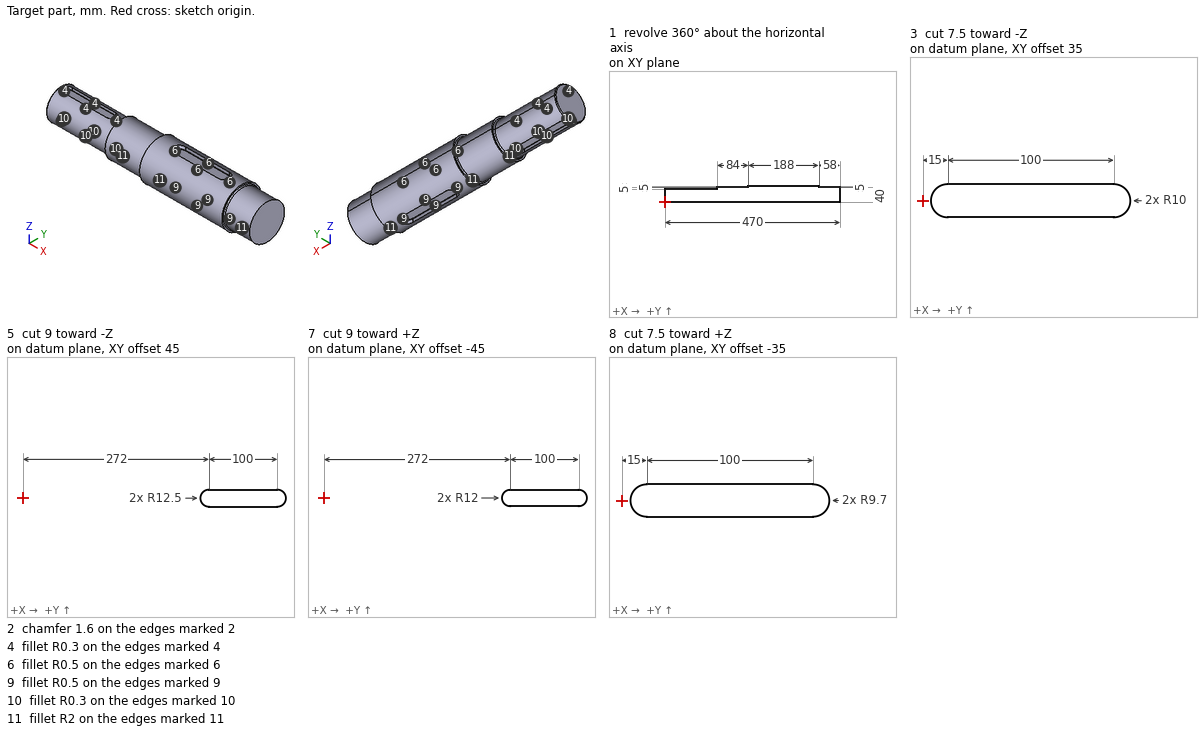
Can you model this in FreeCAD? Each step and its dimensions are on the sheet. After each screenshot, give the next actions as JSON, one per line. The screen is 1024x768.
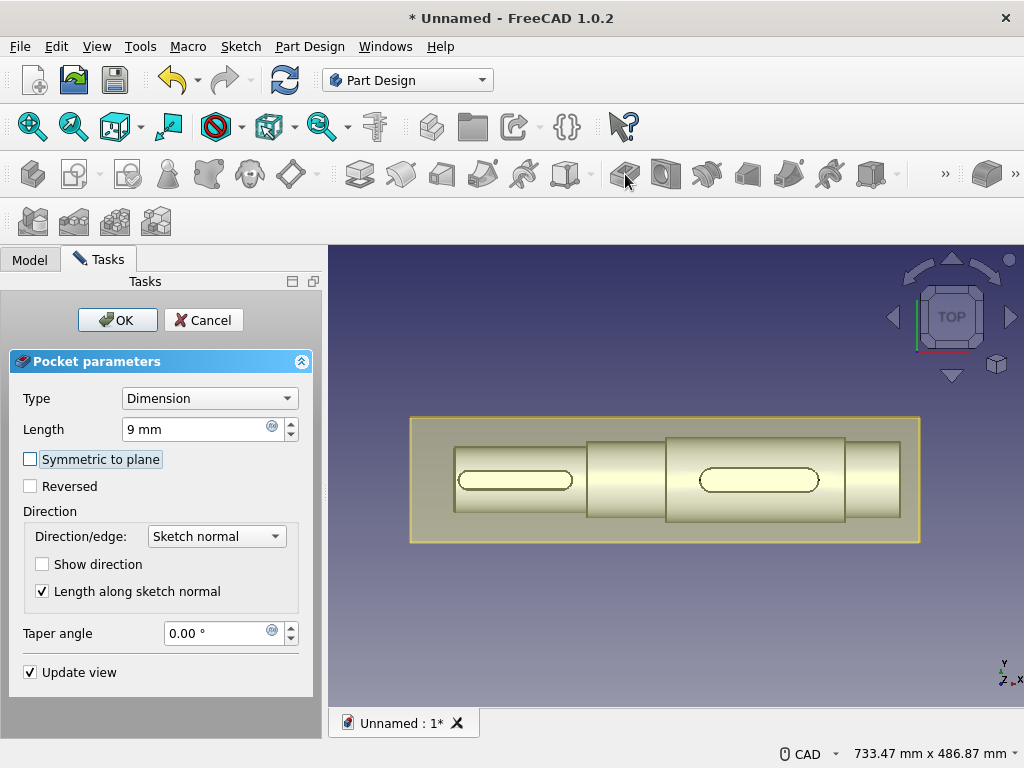
{"action": "left_click", "coordinate": [118, 320]}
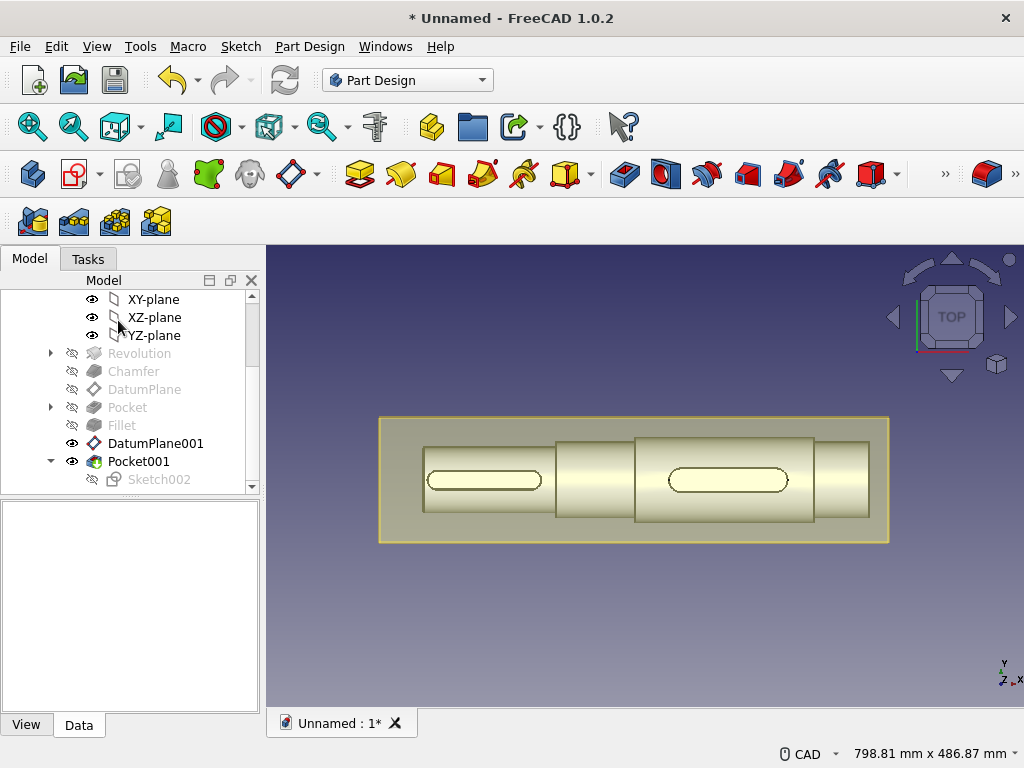
{"action": "left_click", "coordinate": [117, 443]}
{"action": "key", "text": "space"}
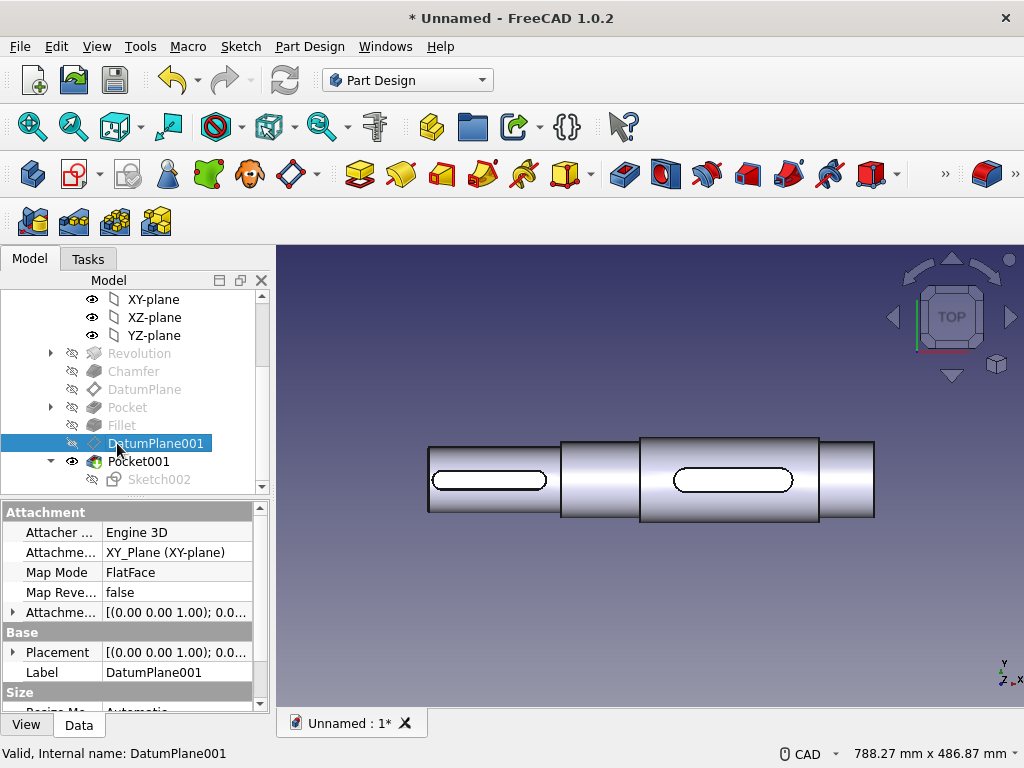
{"action": "left_click", "coordinate": [767, 479]}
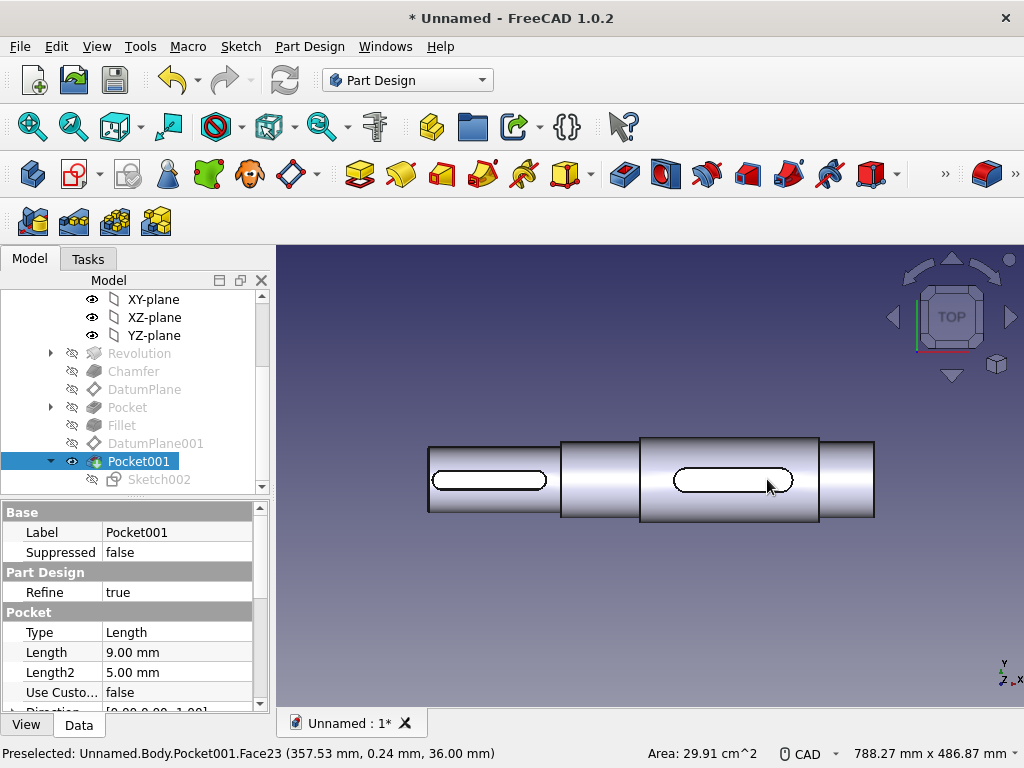
{"action": "left_click", "coordinate": [987, 174]}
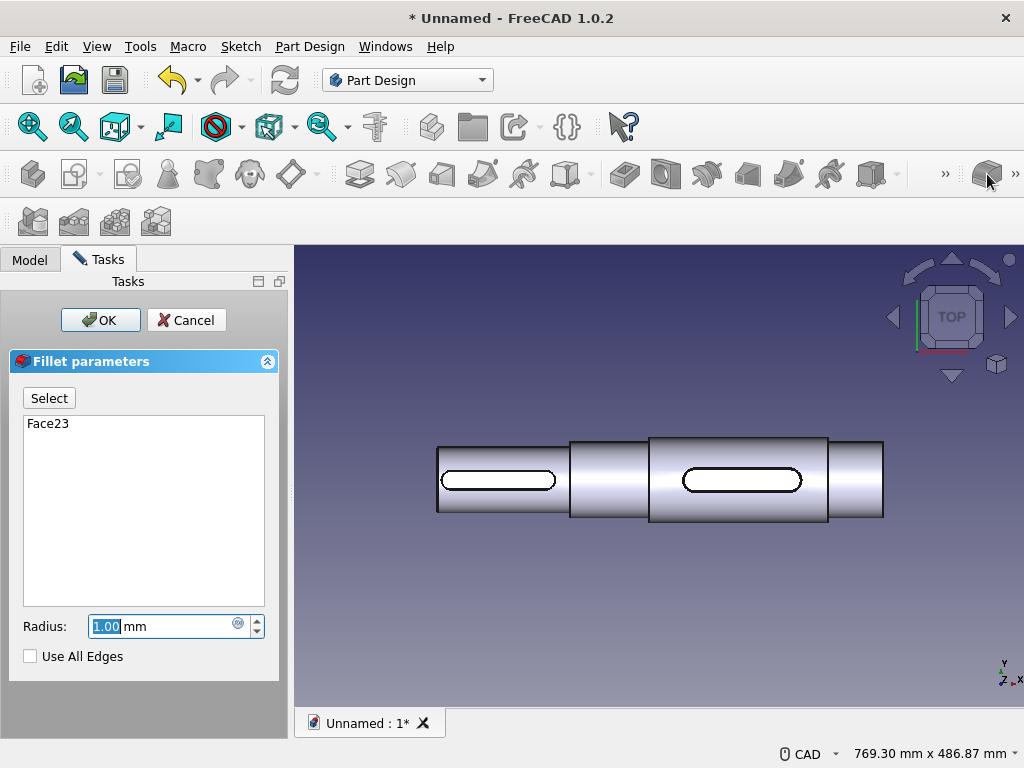
{"action": "type", "text": "0.5"}
{"action": "key", "text": "Tab"}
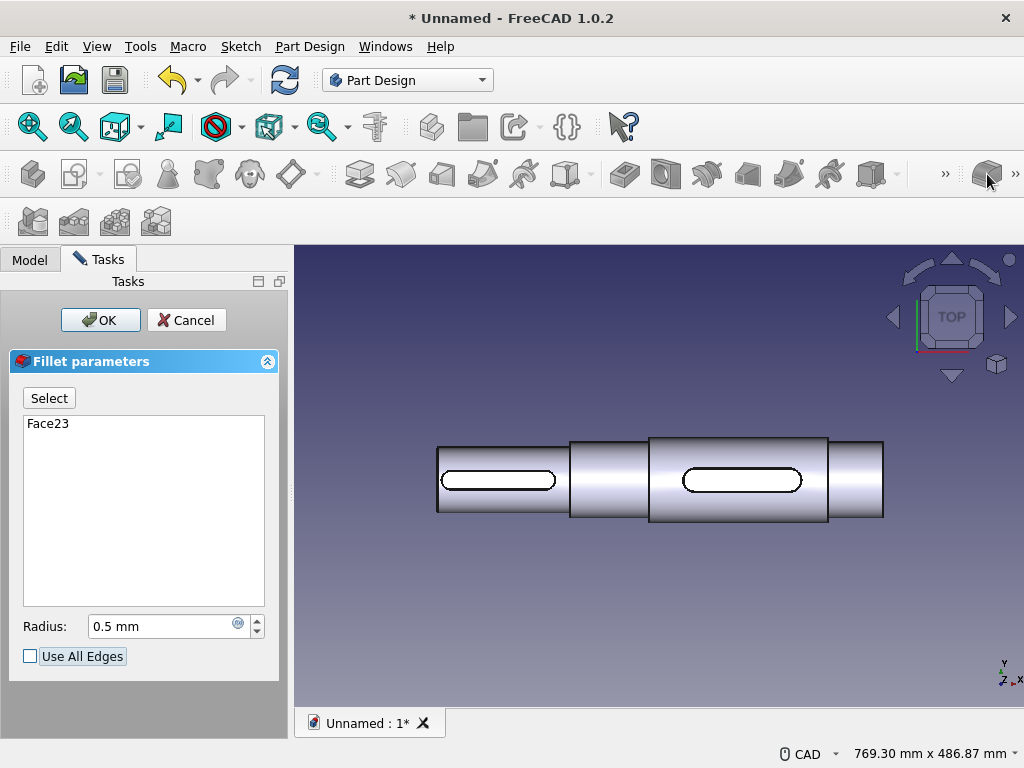
{"action": "left_click", "coordinate": [101, 320]}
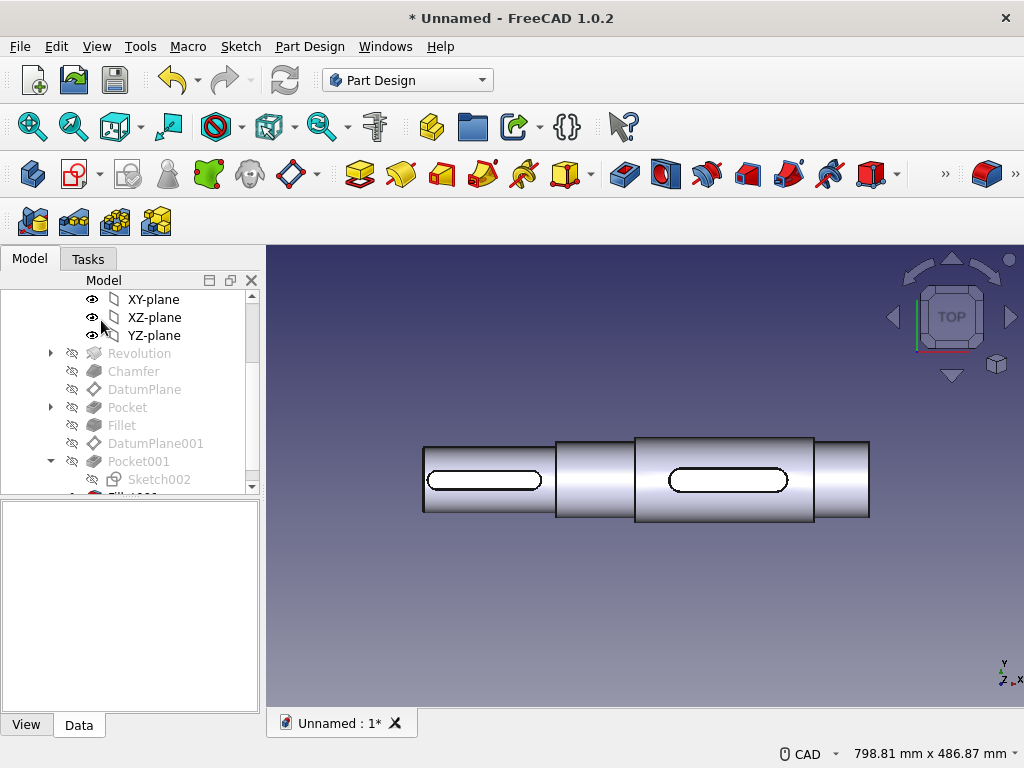
{"action": "scroll", "coordinate": [161, 385], "scroll_direction": "down", "scroll_amount": 3}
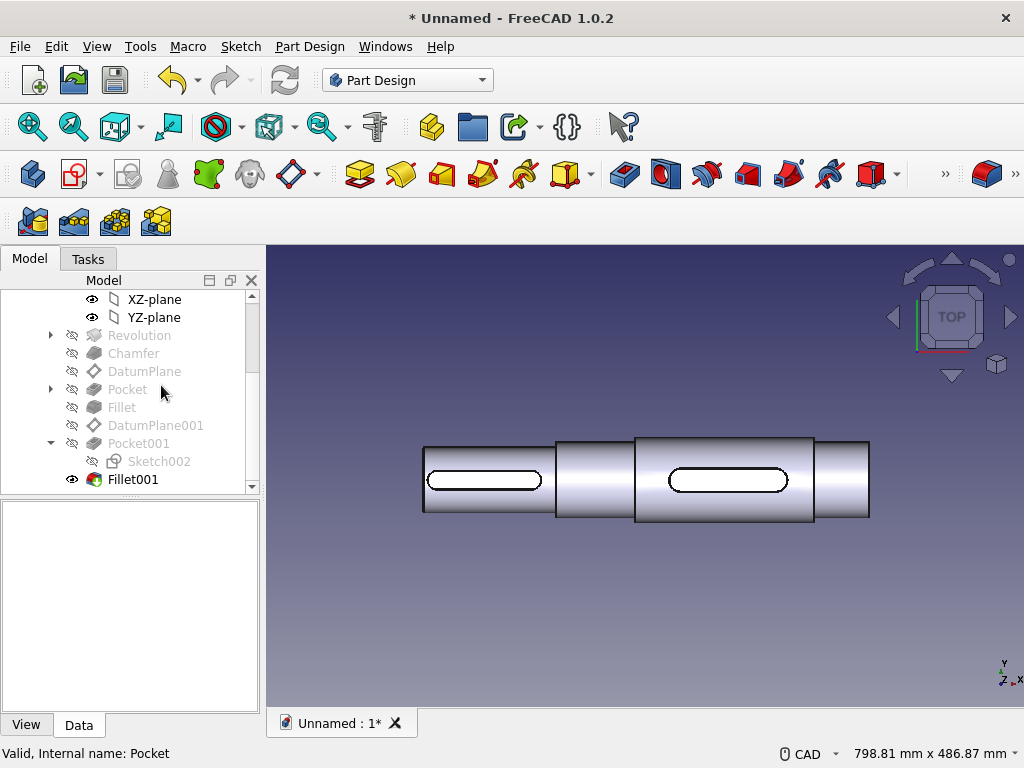
{"action": "scroll", "coordinate": [161, 385], "scroll_direction": "up", "scroll_amount": 15}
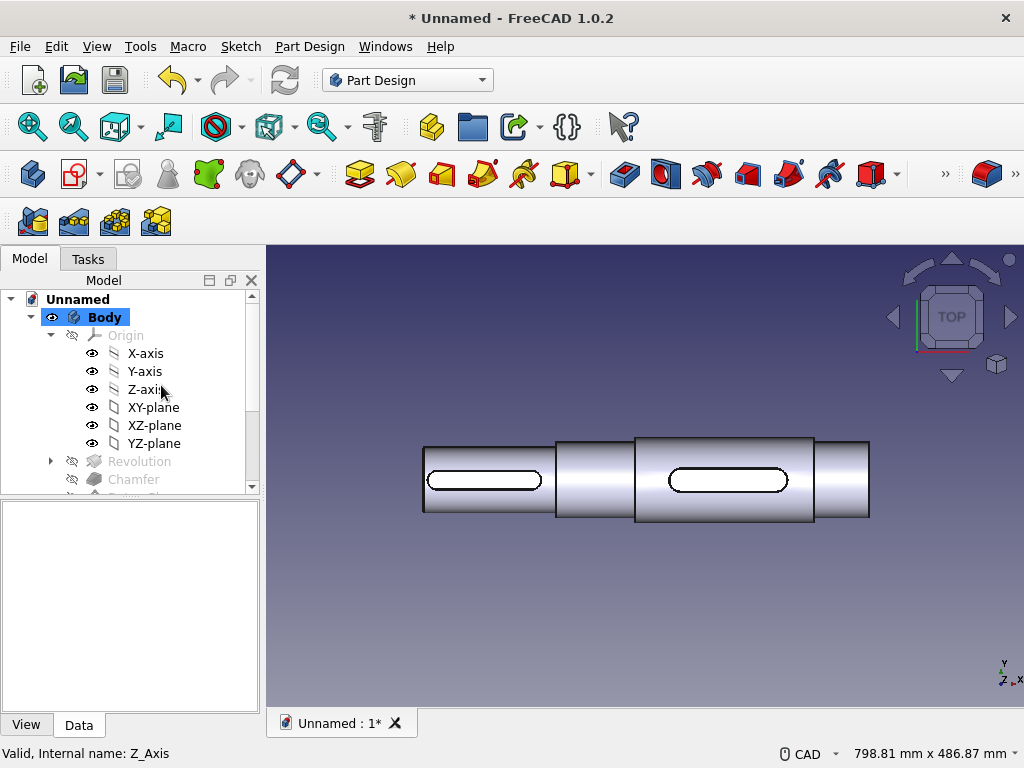
{"action": "left_click", "coordinate": [137, 407]}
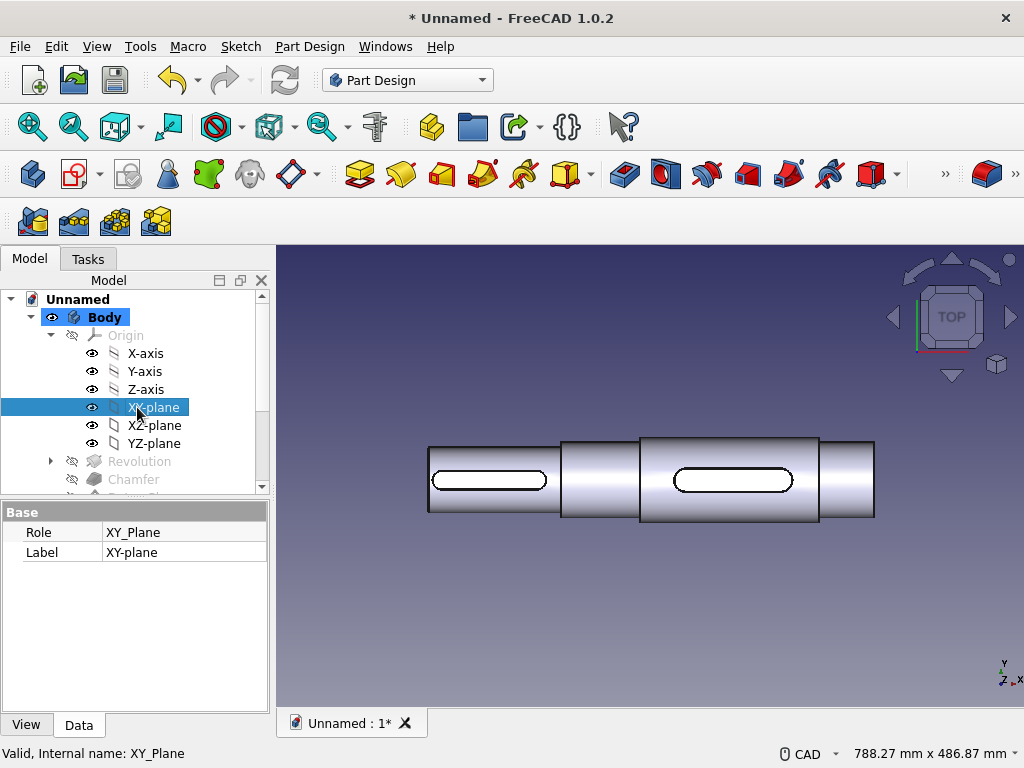
{"action": "left_click", "coordinate": [290, 174]}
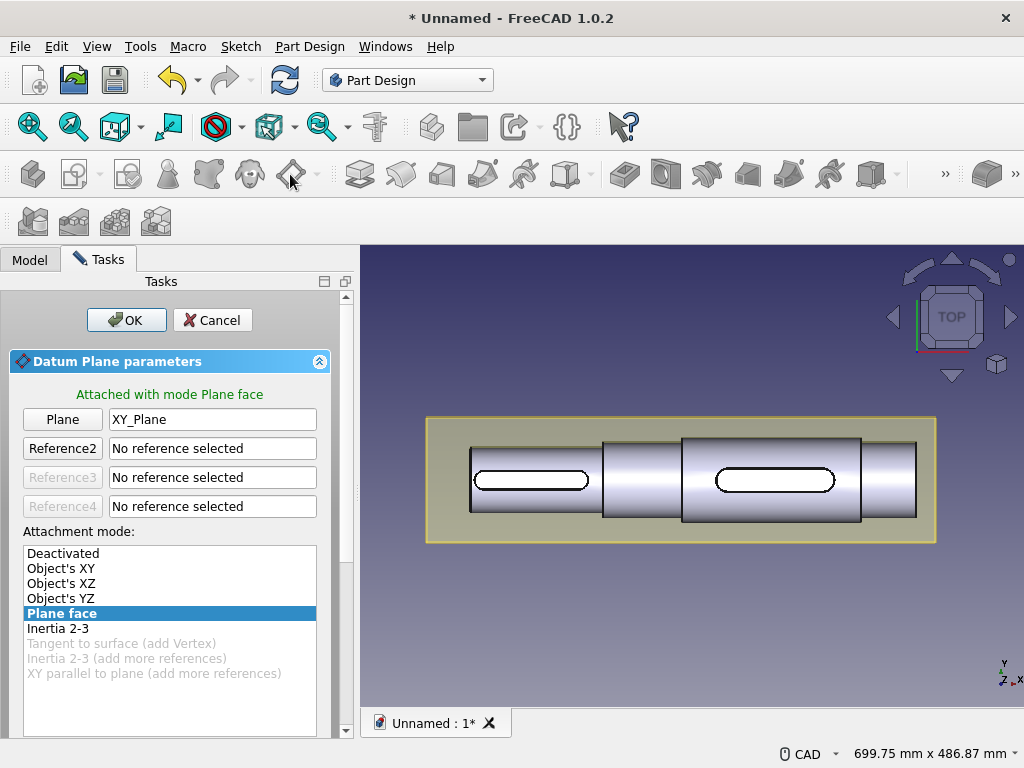
{"action": "scroll", "coordinate": [346, 514], "scroll_direction": "down", "scroll_amount": 4}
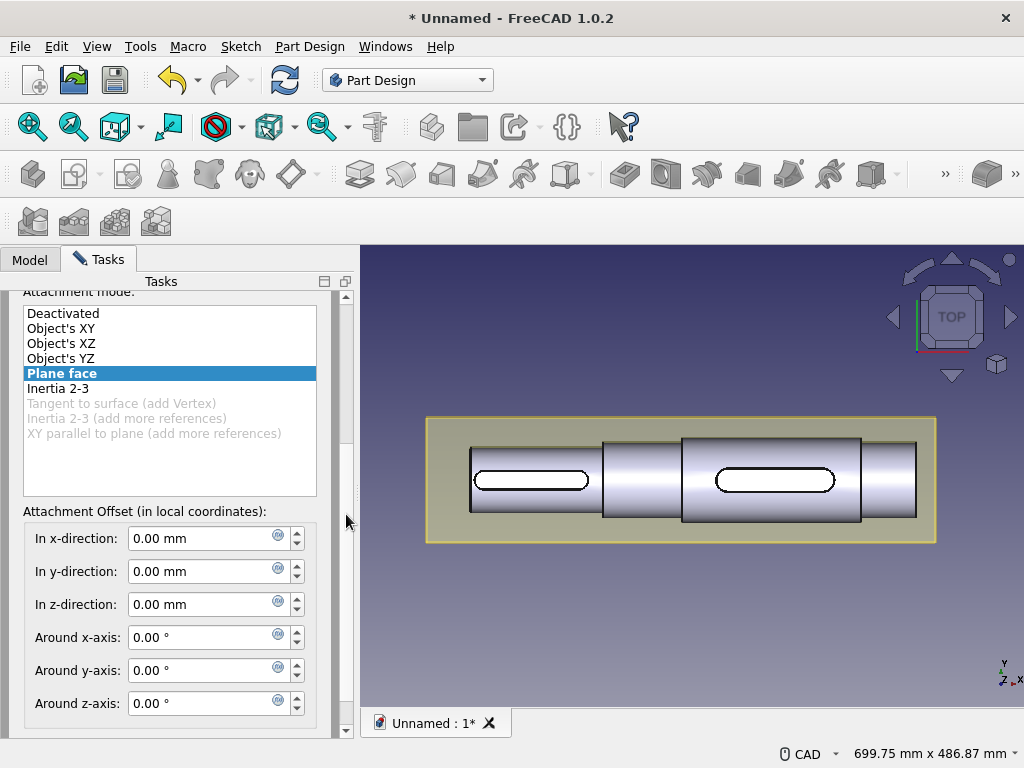
{"action": "triple_click", "coordinate": [210, 604]}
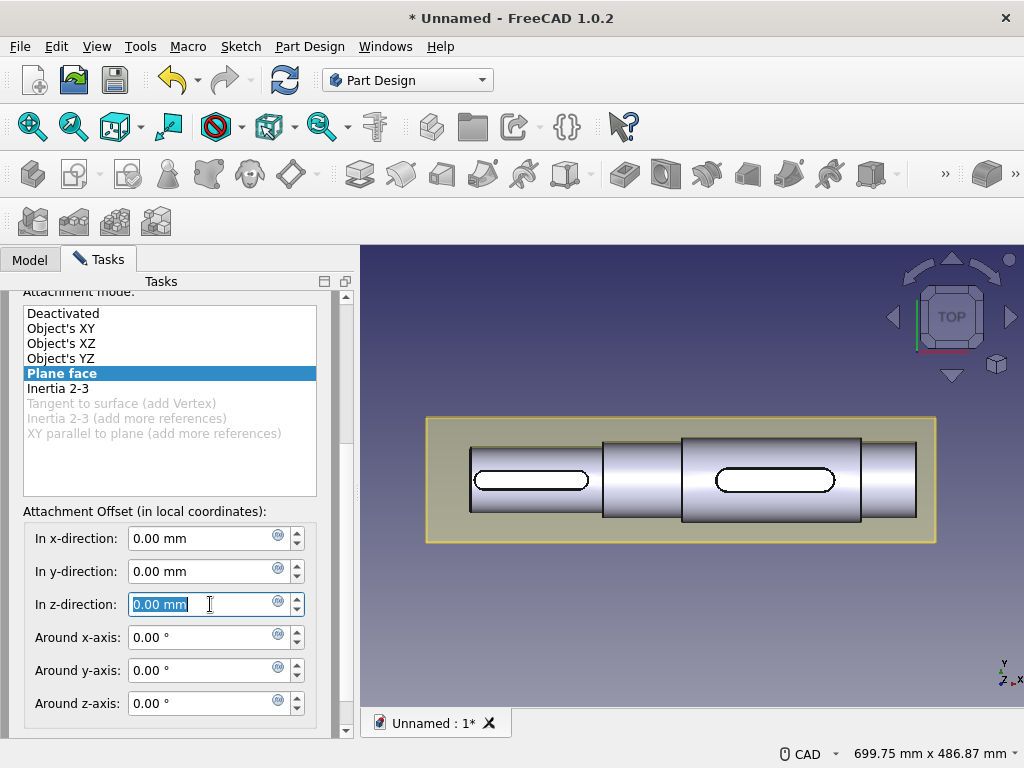
{"action": "type", "text": "-45"}
{"action": "key", "text": "Tab"}